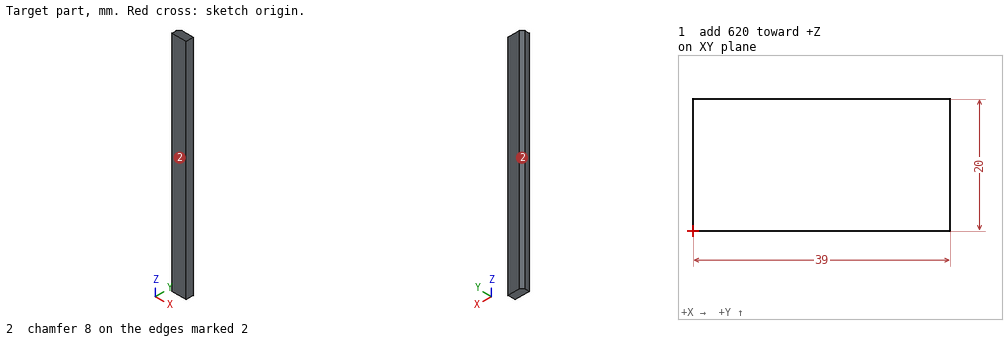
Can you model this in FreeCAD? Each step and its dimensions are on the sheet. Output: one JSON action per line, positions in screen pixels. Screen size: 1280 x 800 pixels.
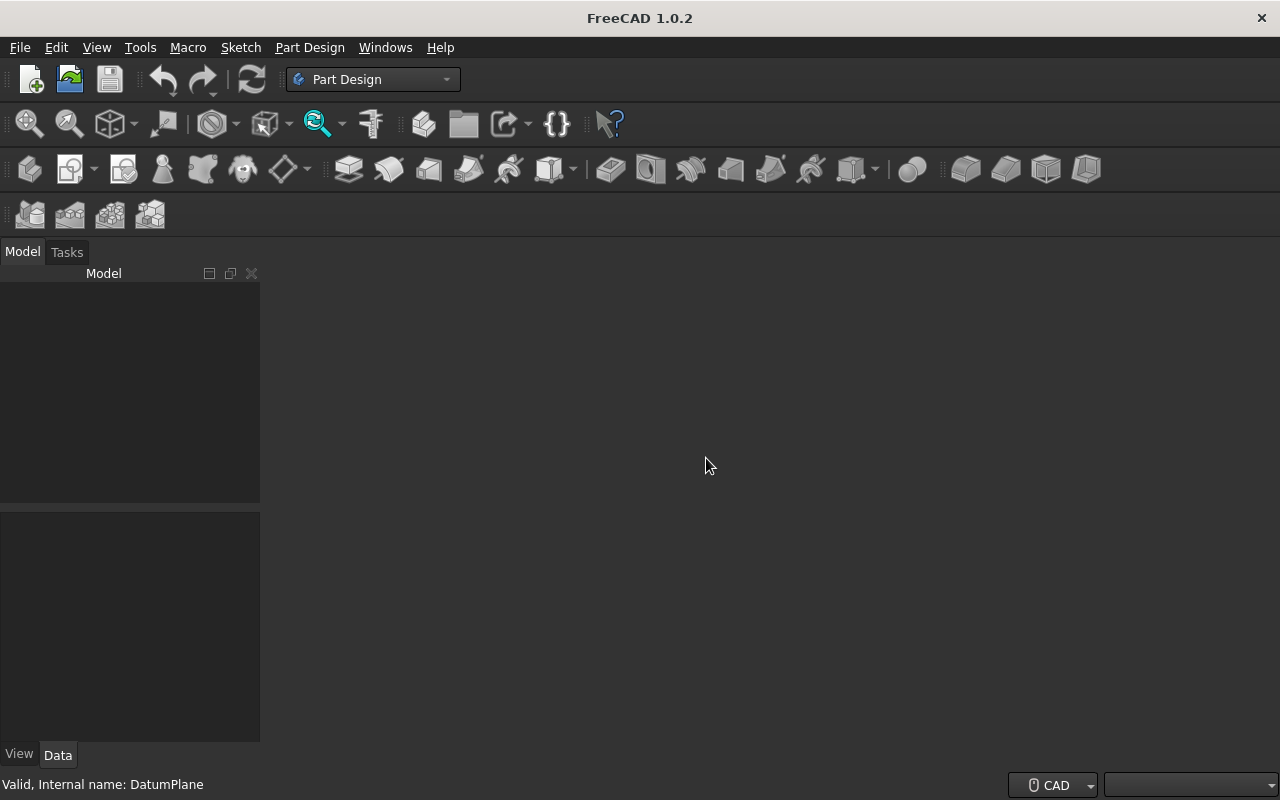
{"action": "key", "text": "ctrl+n"}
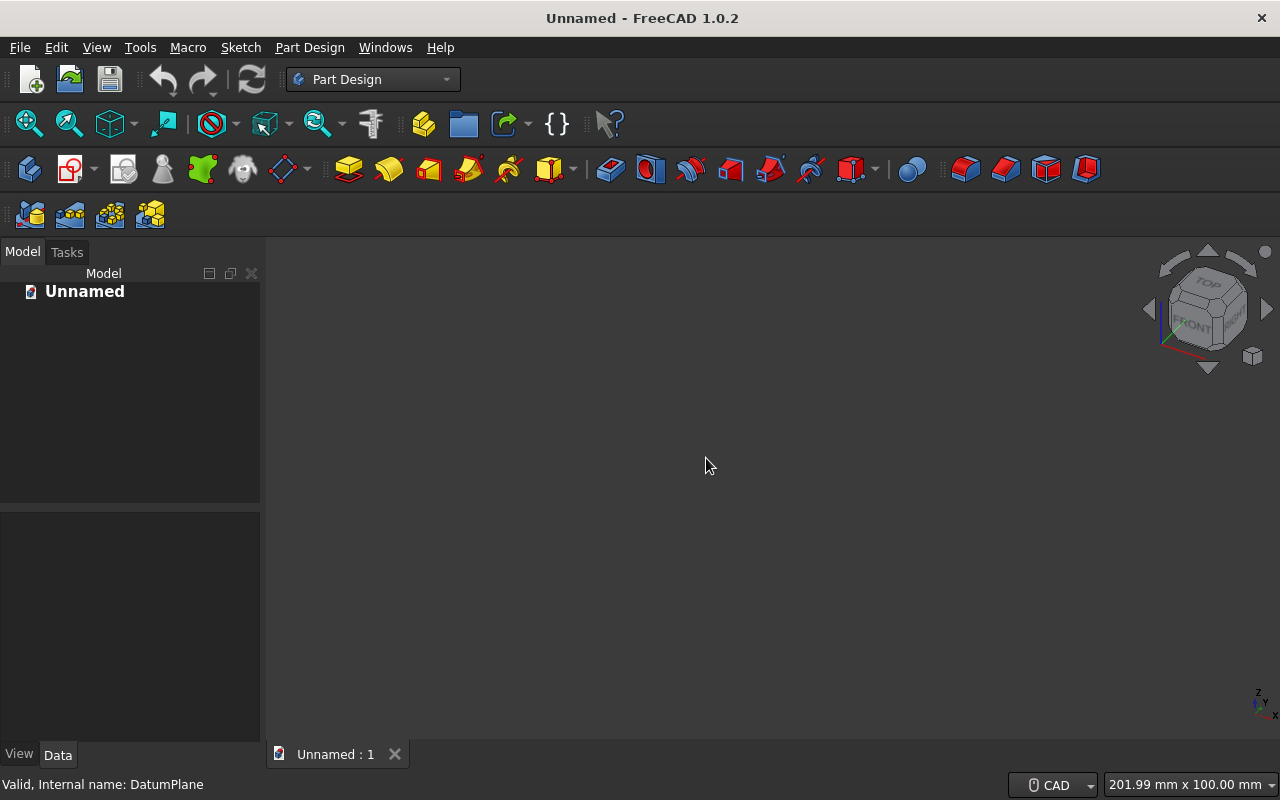
{"action": "left_click", "coordinate": [70, 170]}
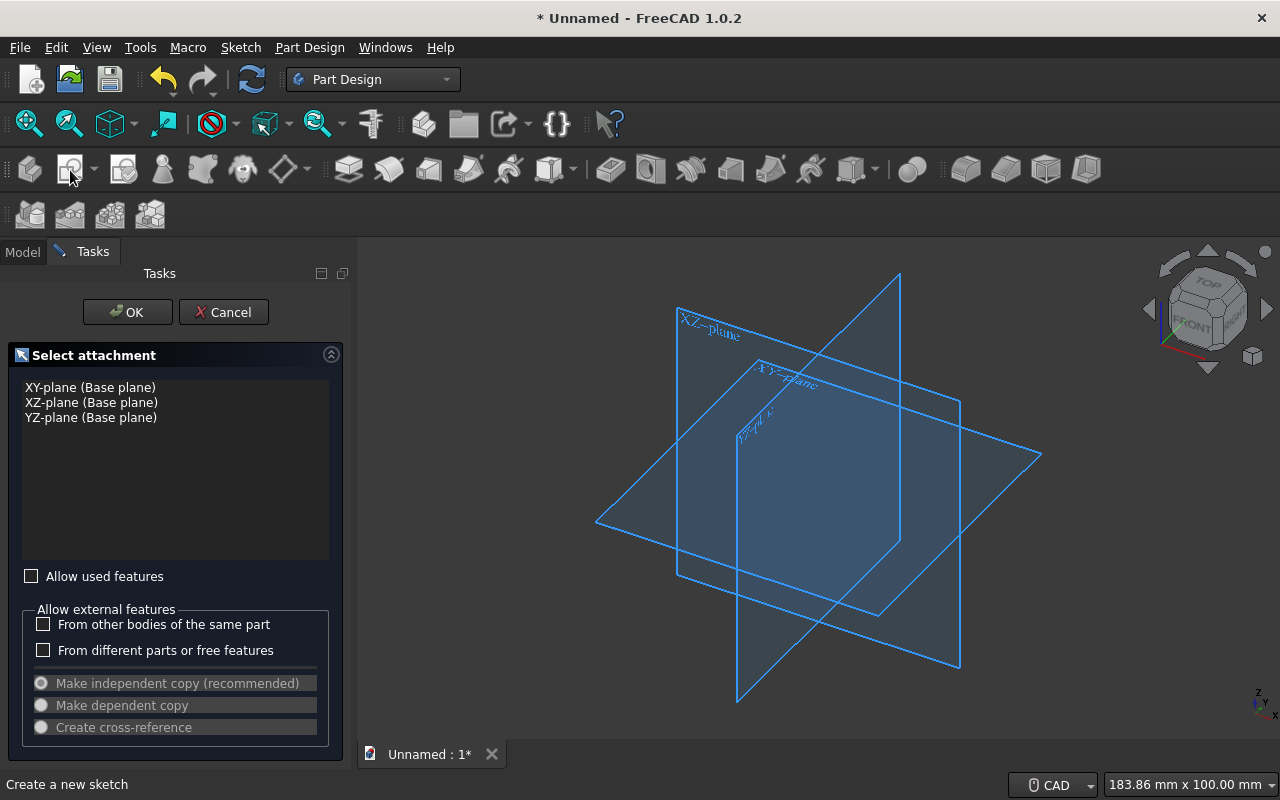
{"action": "left_click", "coordinate": [82, 388]}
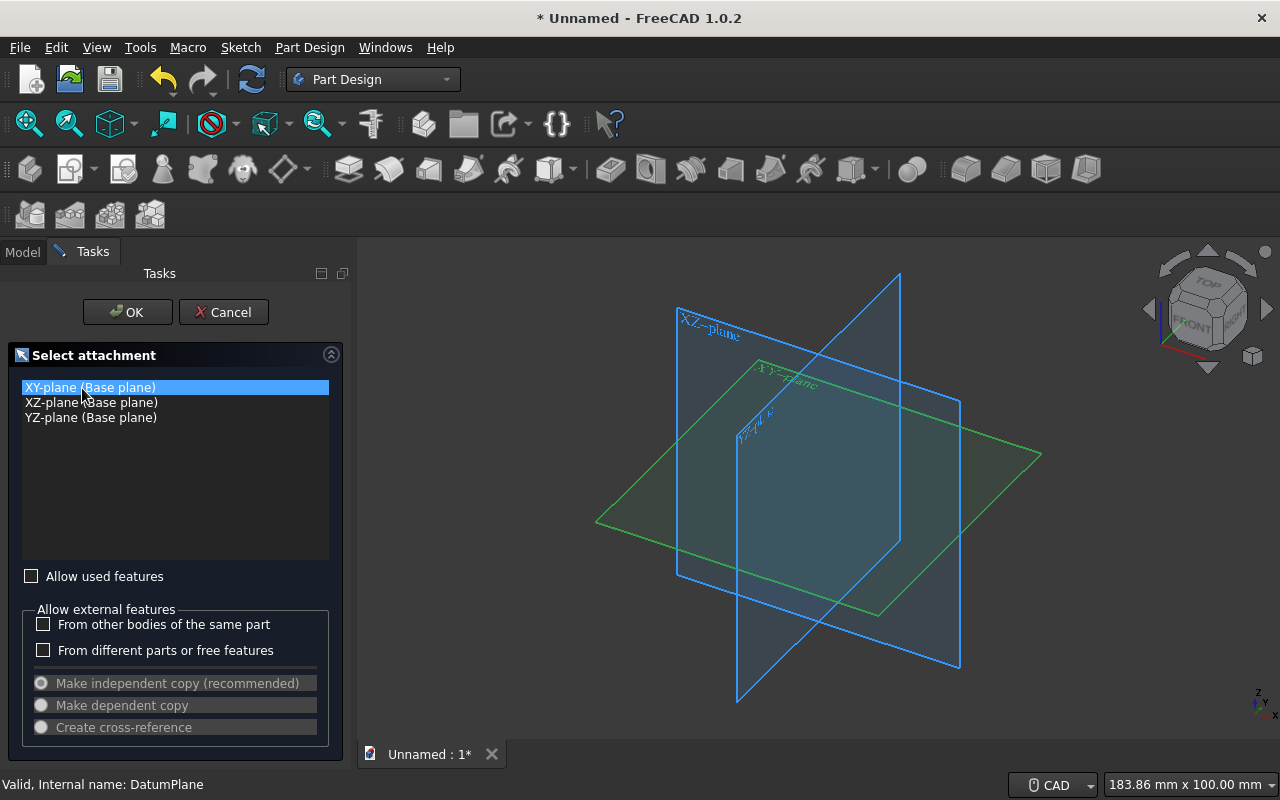
{"action": "left_click", "coordinate": [128, 312]}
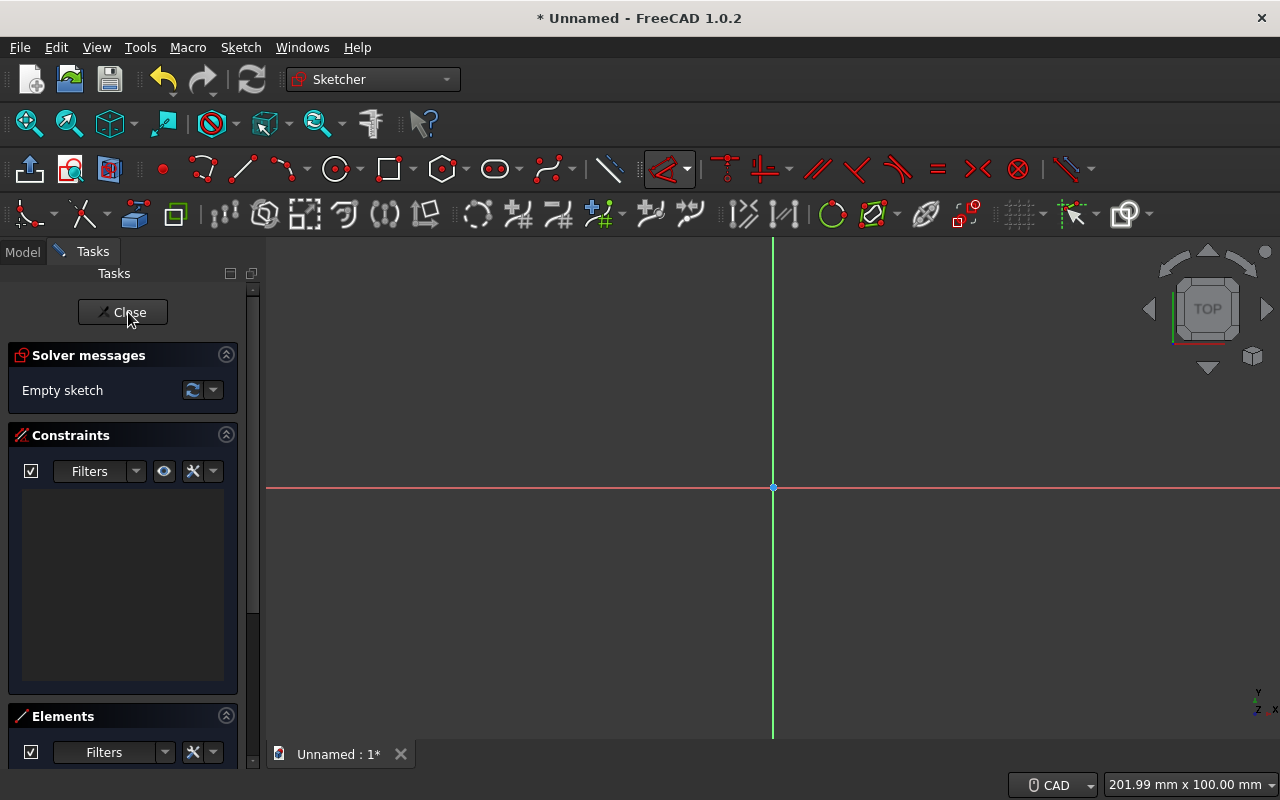
{"action": "scroll", "coordinate": [968, 409], "scroll_direction": "up", "scroll_amount": 5}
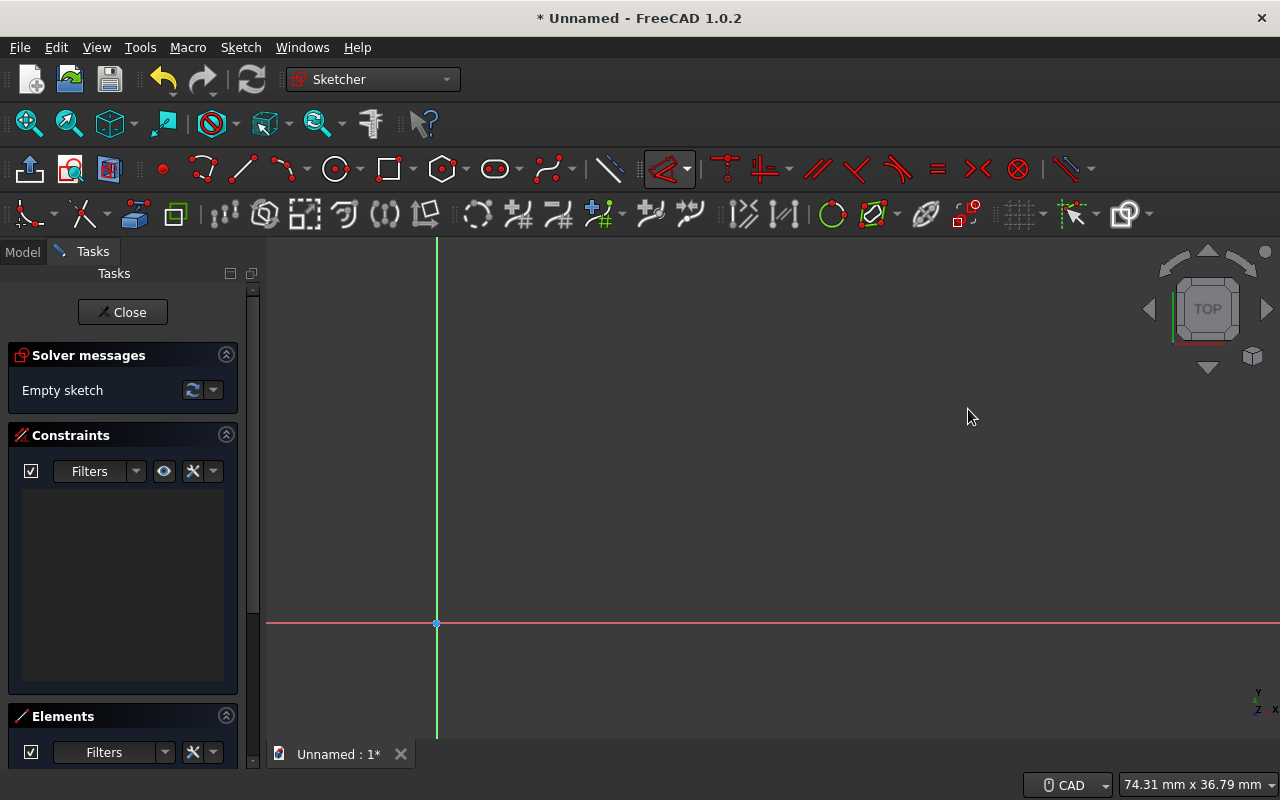
{"action": "key", "text": "g r"}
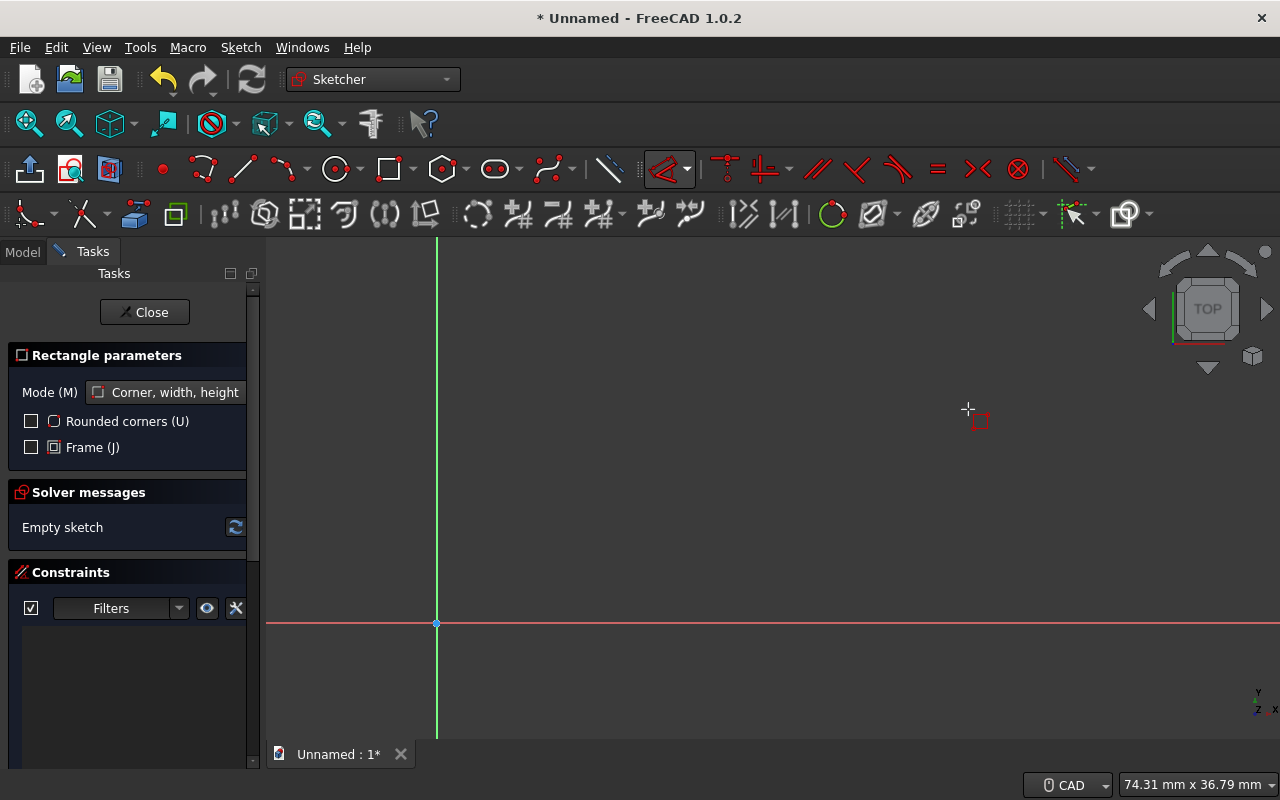
{"action": "left_click", "coordinate": [437, 623]}
{"action": "left_click", "coordinate": [969, 350]}
{"action": "key", "text": "Escape"}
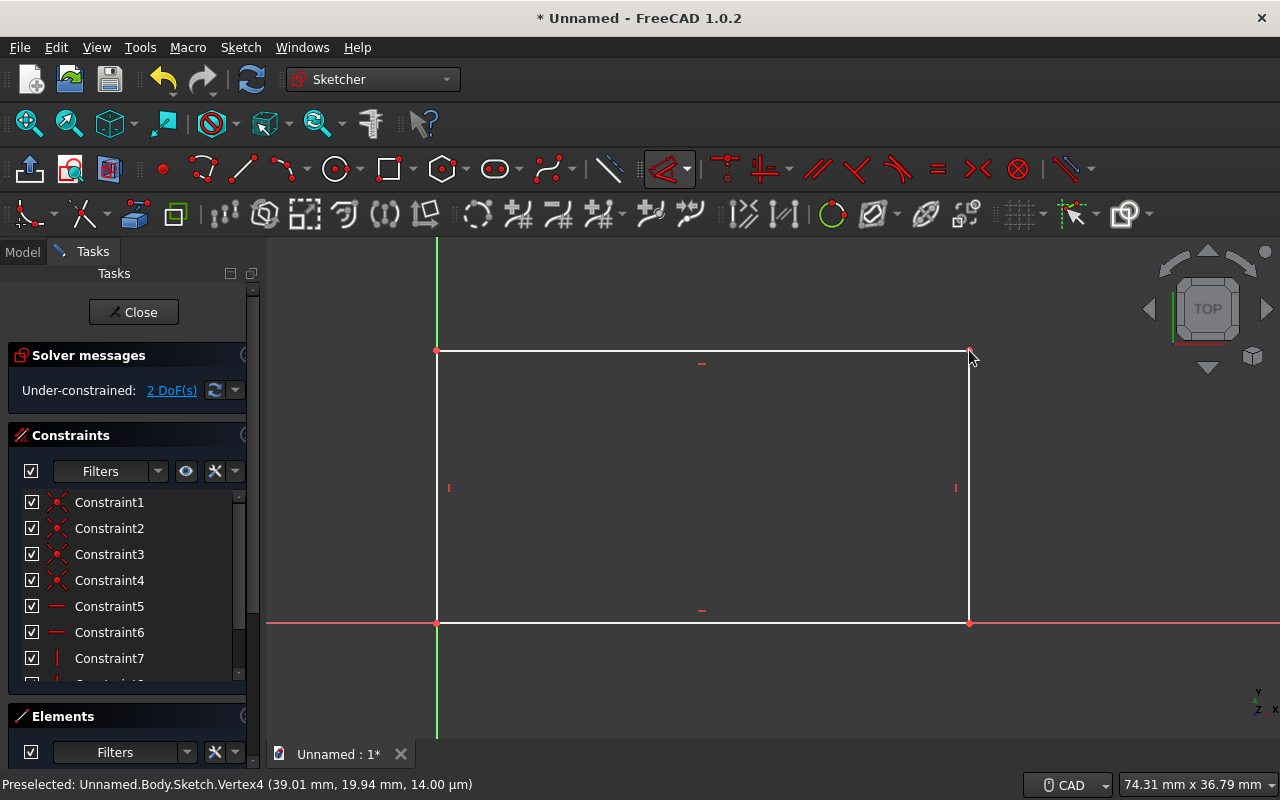
{"action": "left_click", "coordinate": [664, 170]}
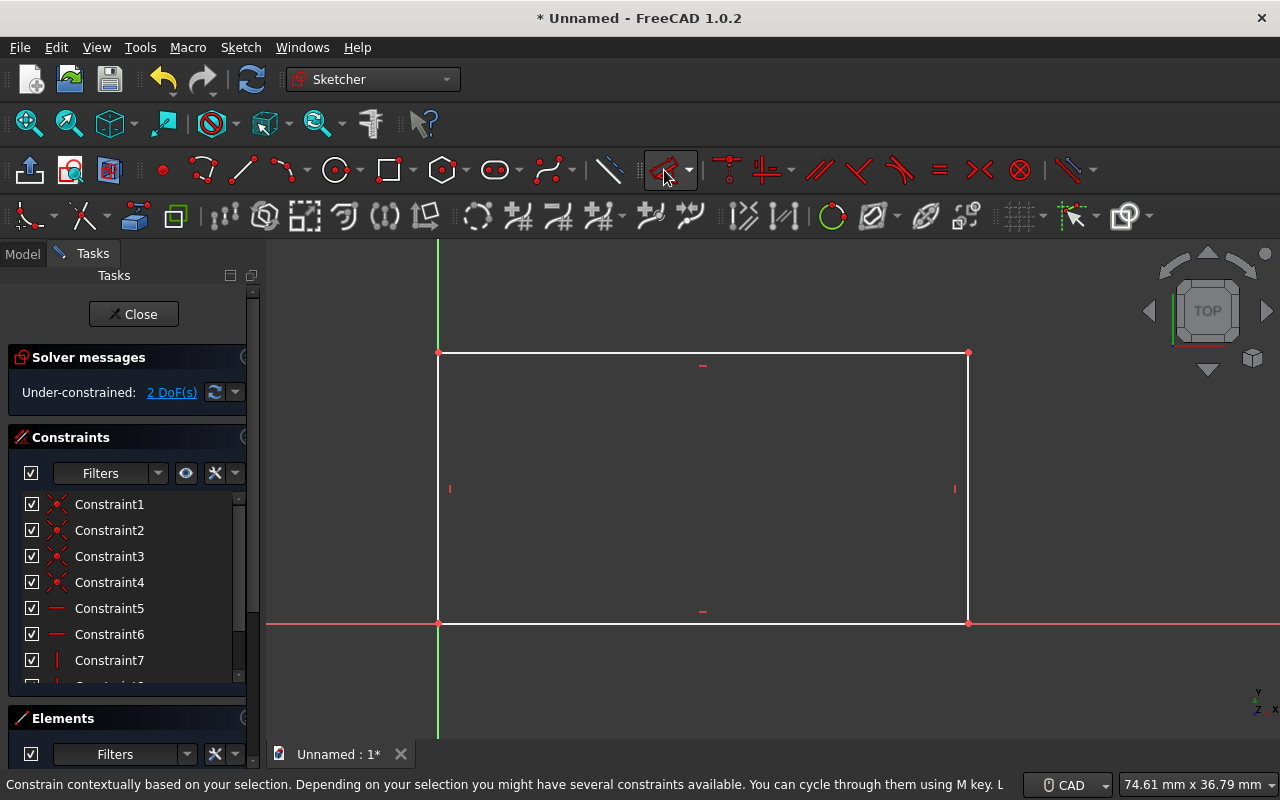
{"action": "left_click", "coordinate": [597, 624]}
{"action": "left_click", "coordinate": [703, 658]}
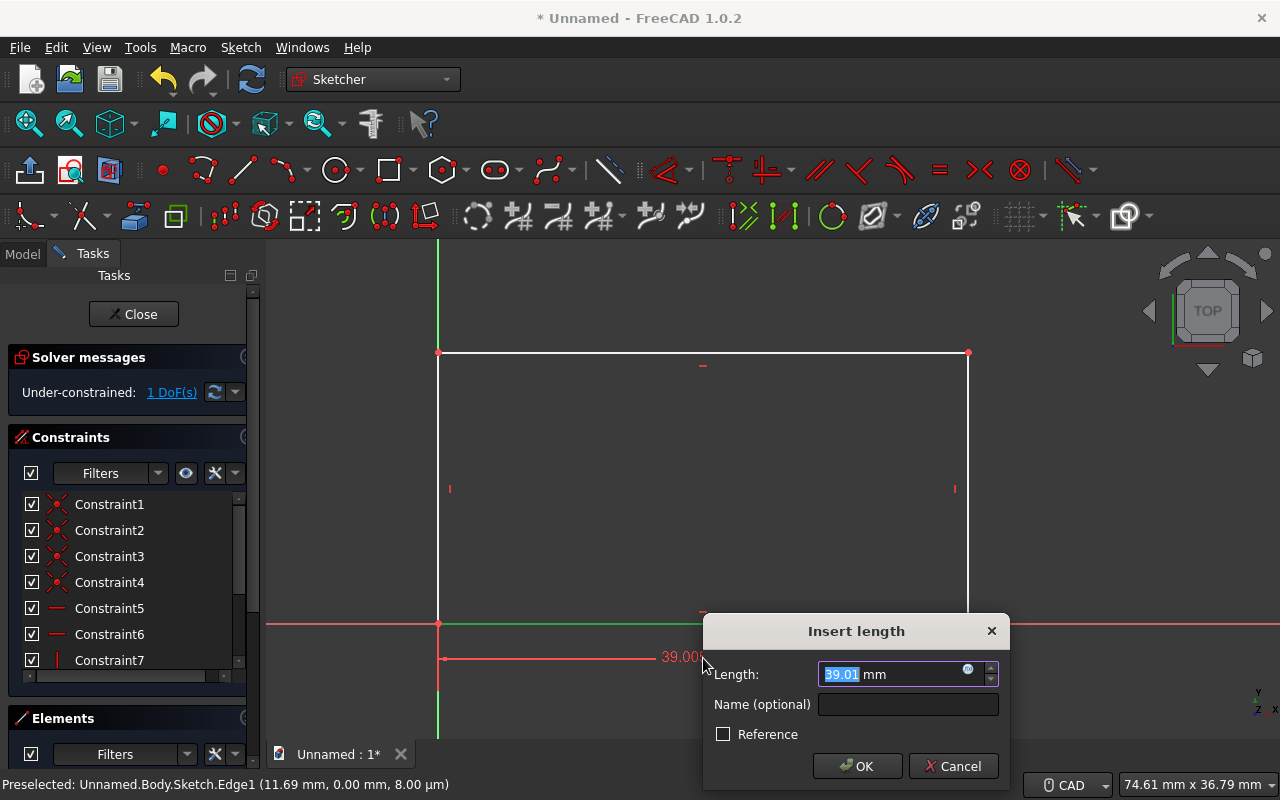
{"action": "type", "text": "39"}
{"action": "key", "text": "Return"}